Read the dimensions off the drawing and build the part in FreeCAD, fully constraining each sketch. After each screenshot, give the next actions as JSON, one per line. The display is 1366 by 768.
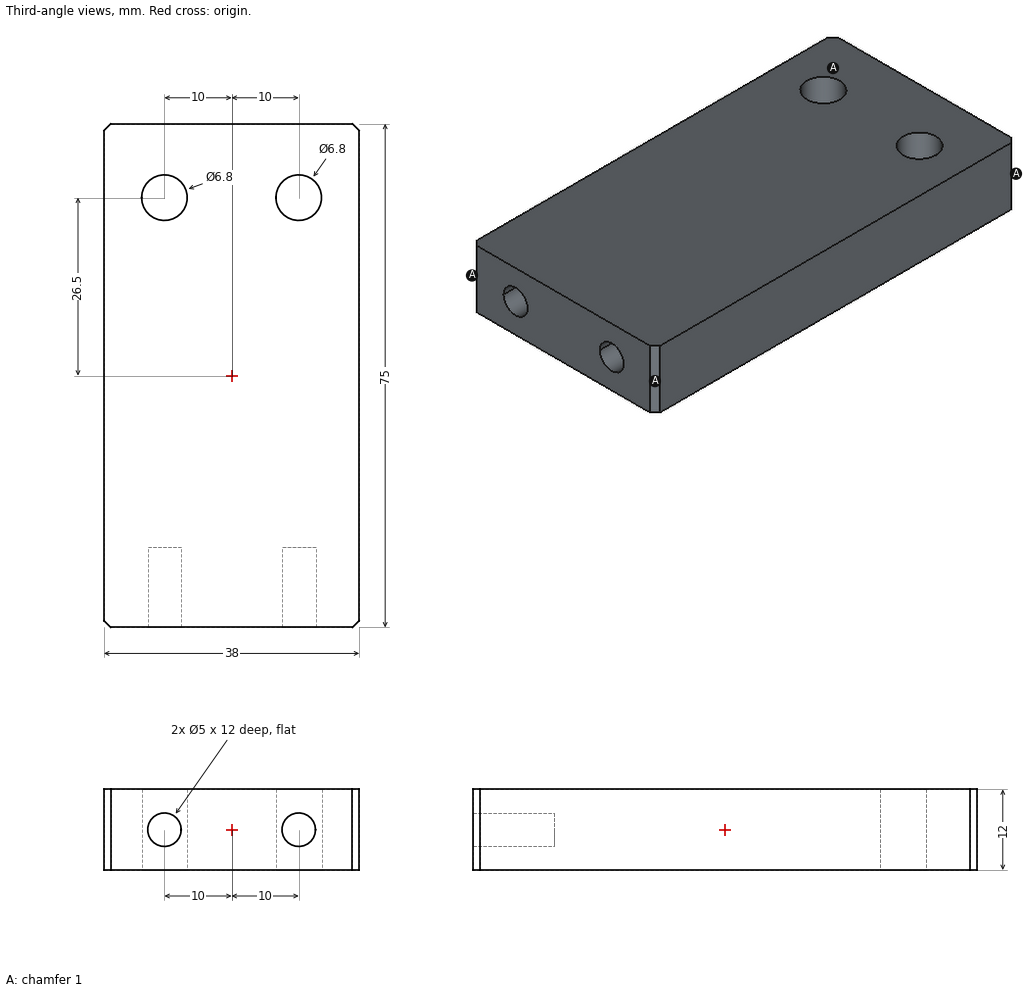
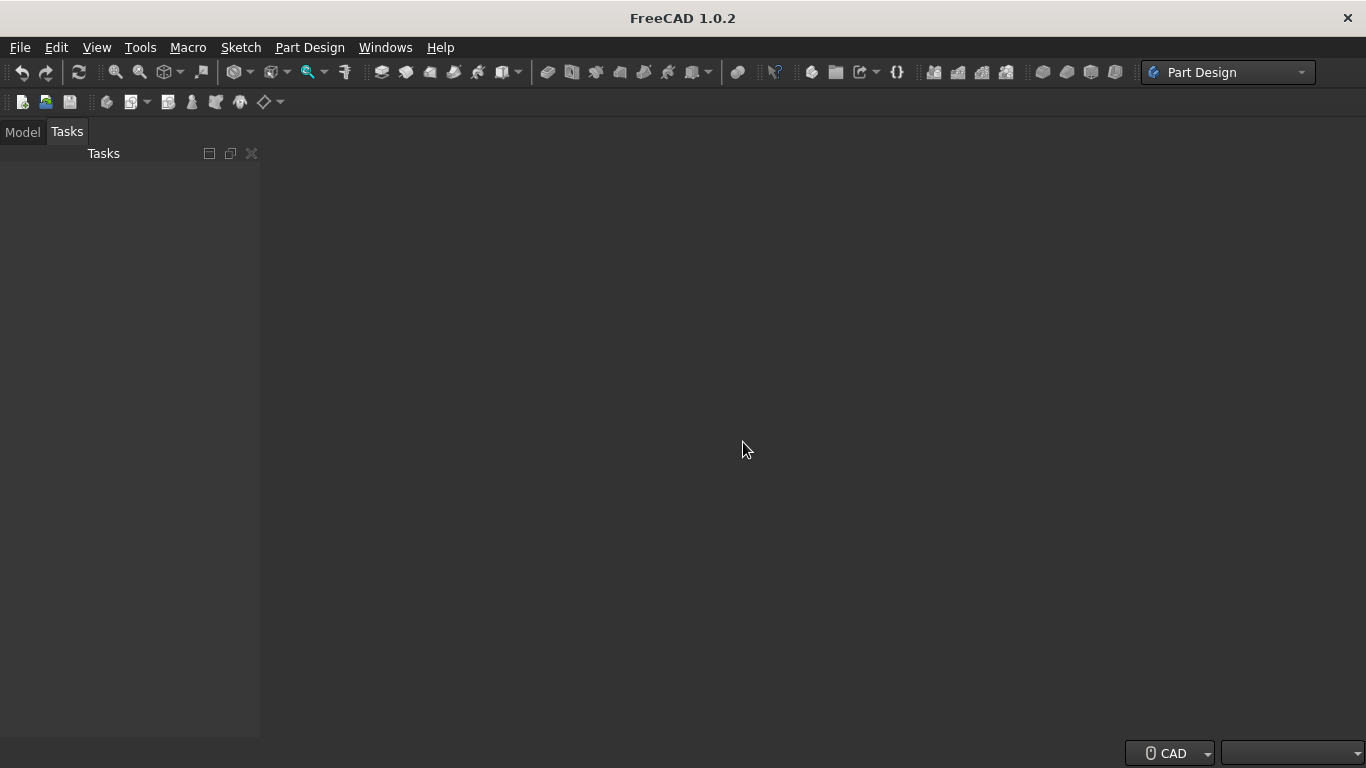
{"action": "key", "text": "ctrl+n"}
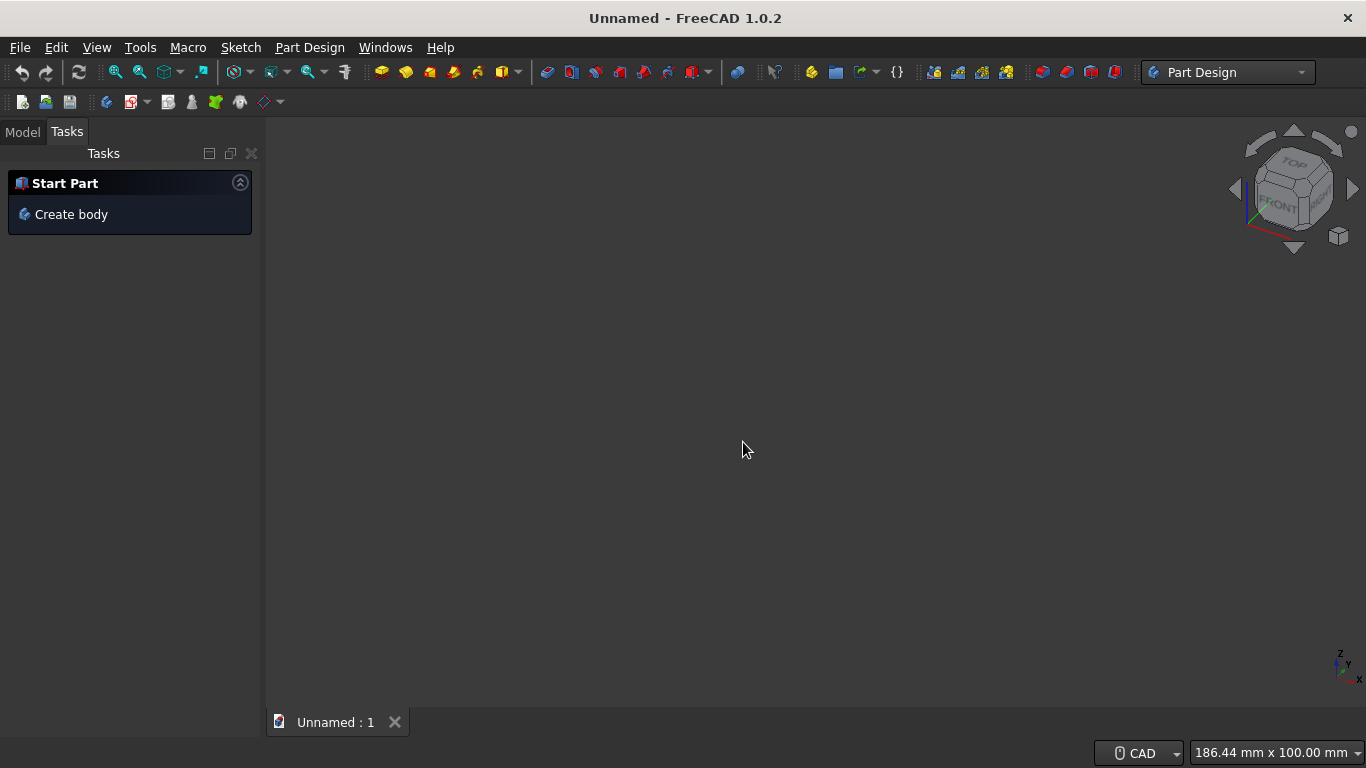
{"action": "left_click", "coordinate": [132, 102]}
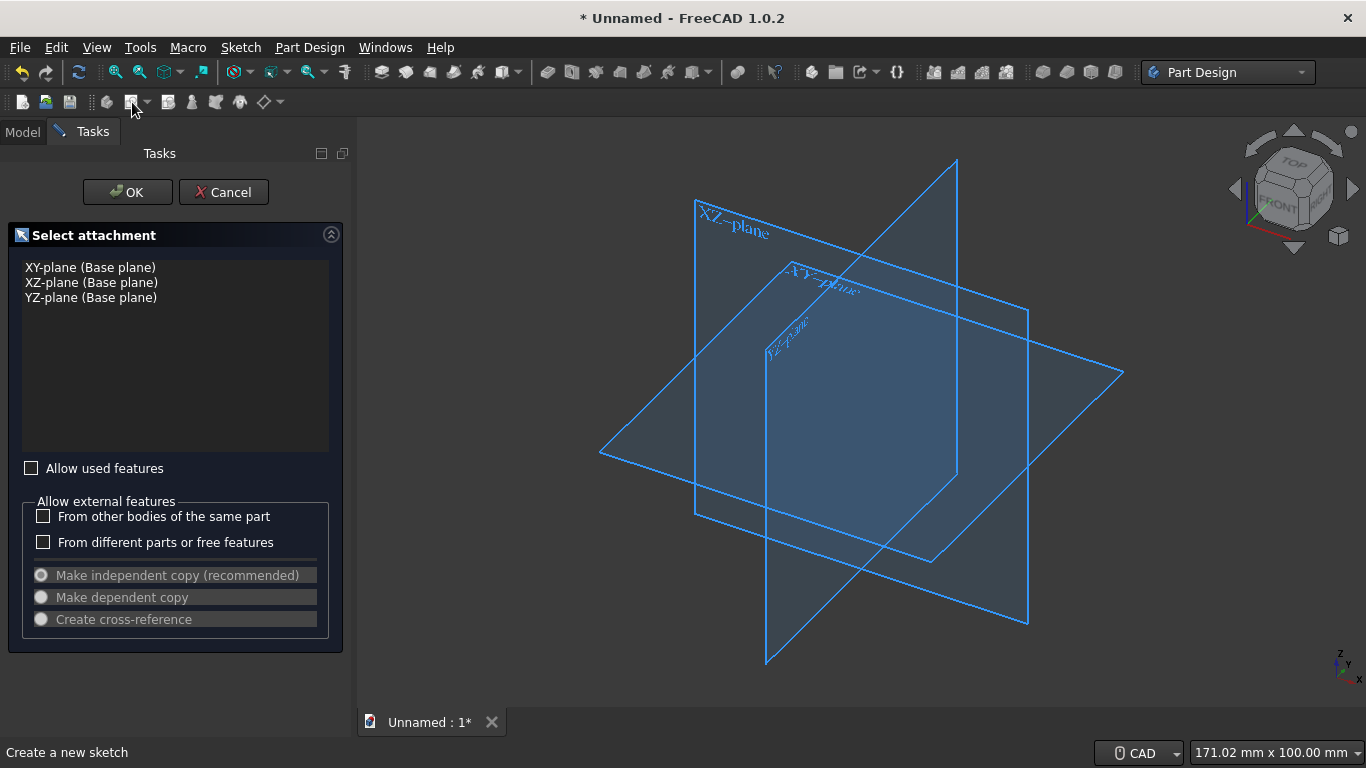
{"action": "left_click", "coordinate": [82, 268]}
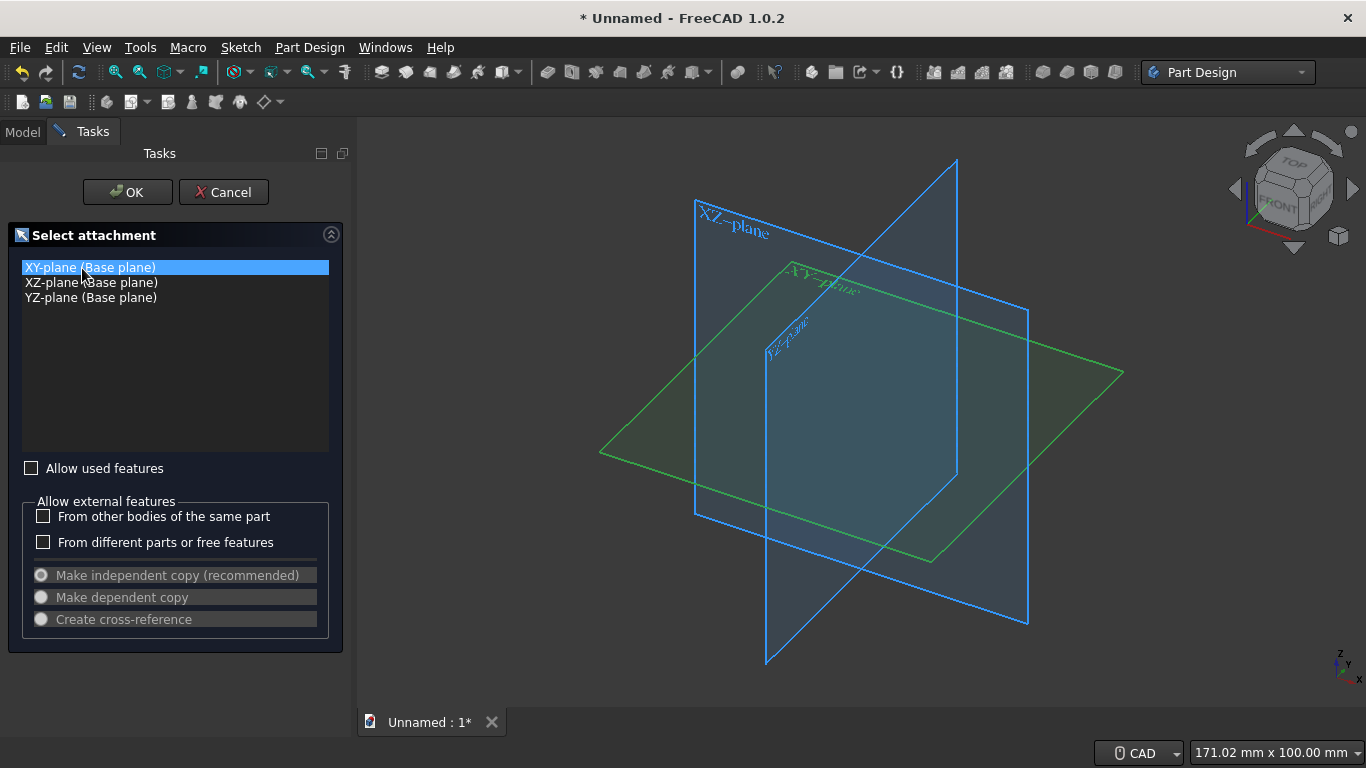
{"action": "left_click", "coordinate": [128, 192]}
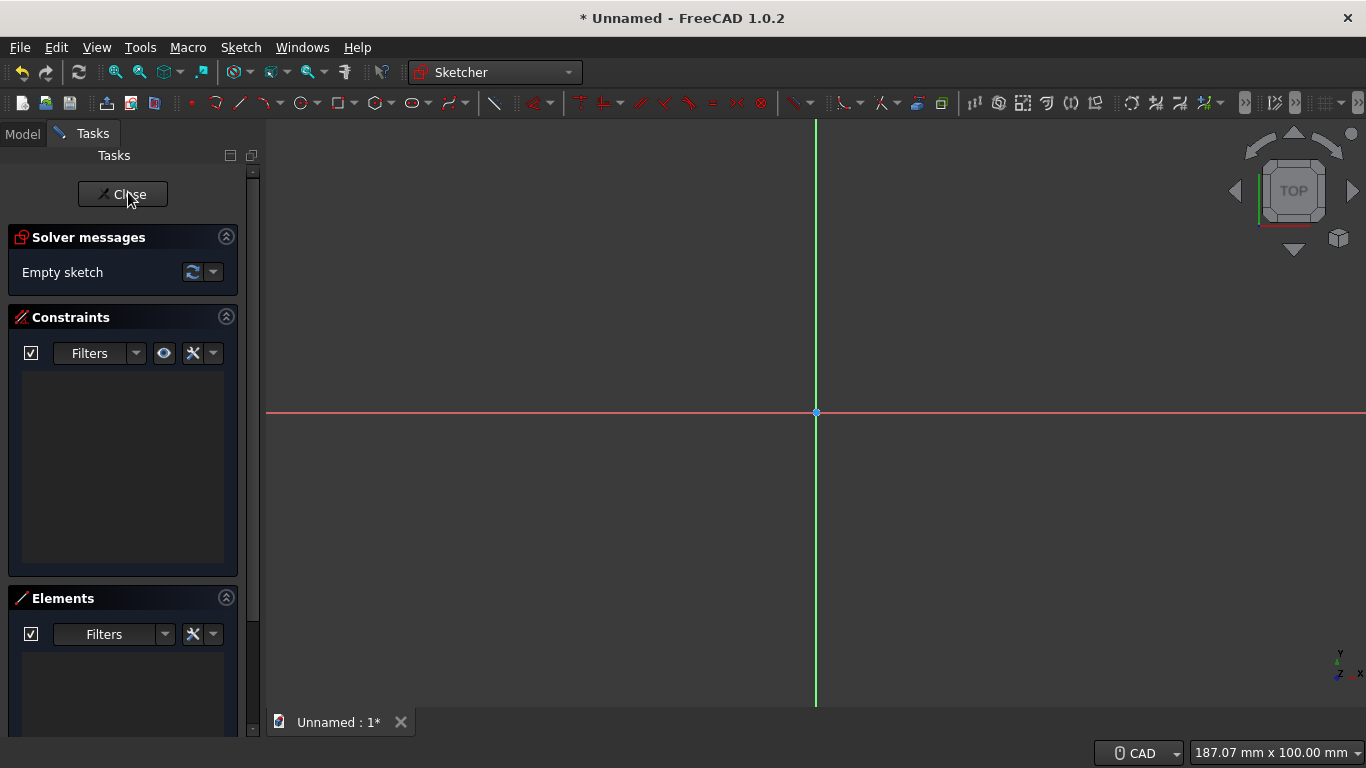
{"action": "key", "text": "g v"}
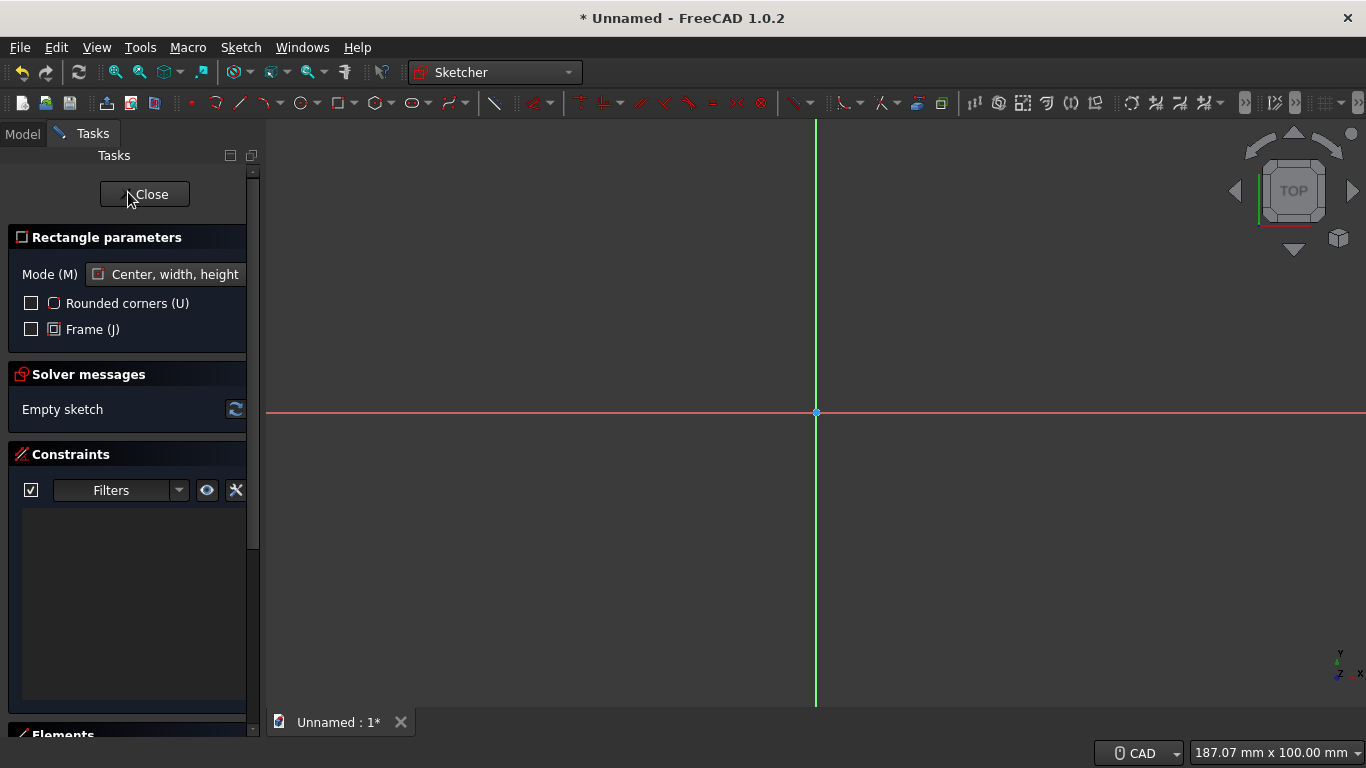
{"action": "left_click", "coordinate": [816, 413]}
{"action": "mouse_move", "coordinate": [928, 192]}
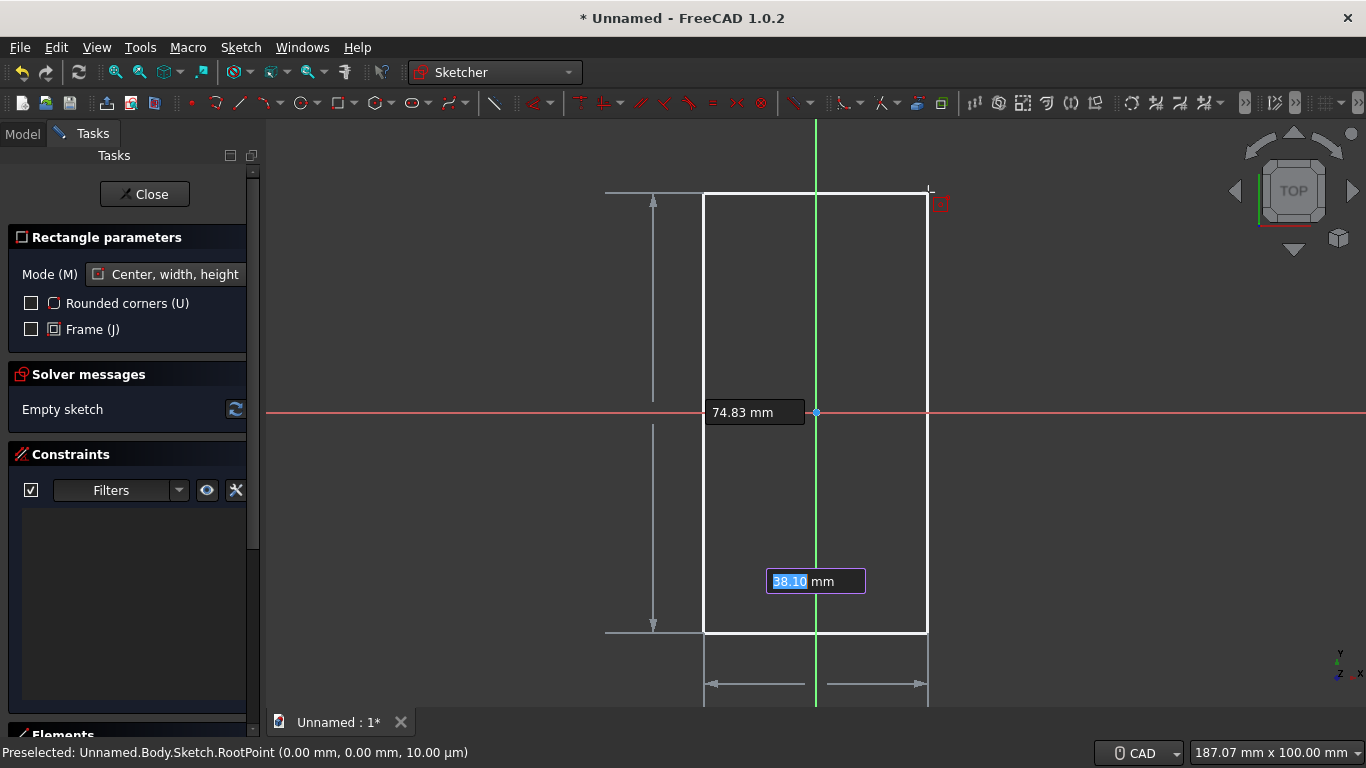
{"action": "type", "text": "38"}
{"action": "key", "text": "Tab"}
{"action": "type", "text": "75"}
{"action": "key", "text": "Return"}
{"action": "key", "text": "Escape"}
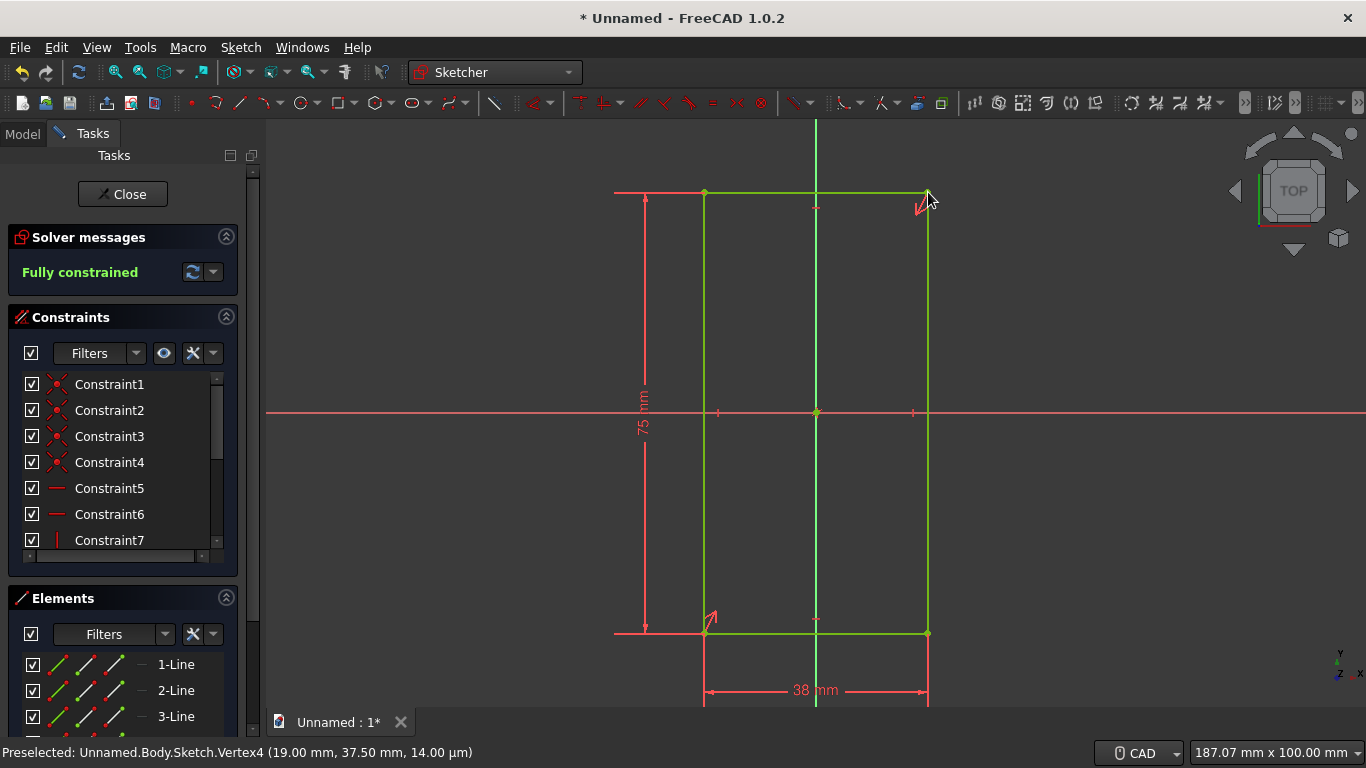
{"action": "left_click", "coordinate": [123, 194]}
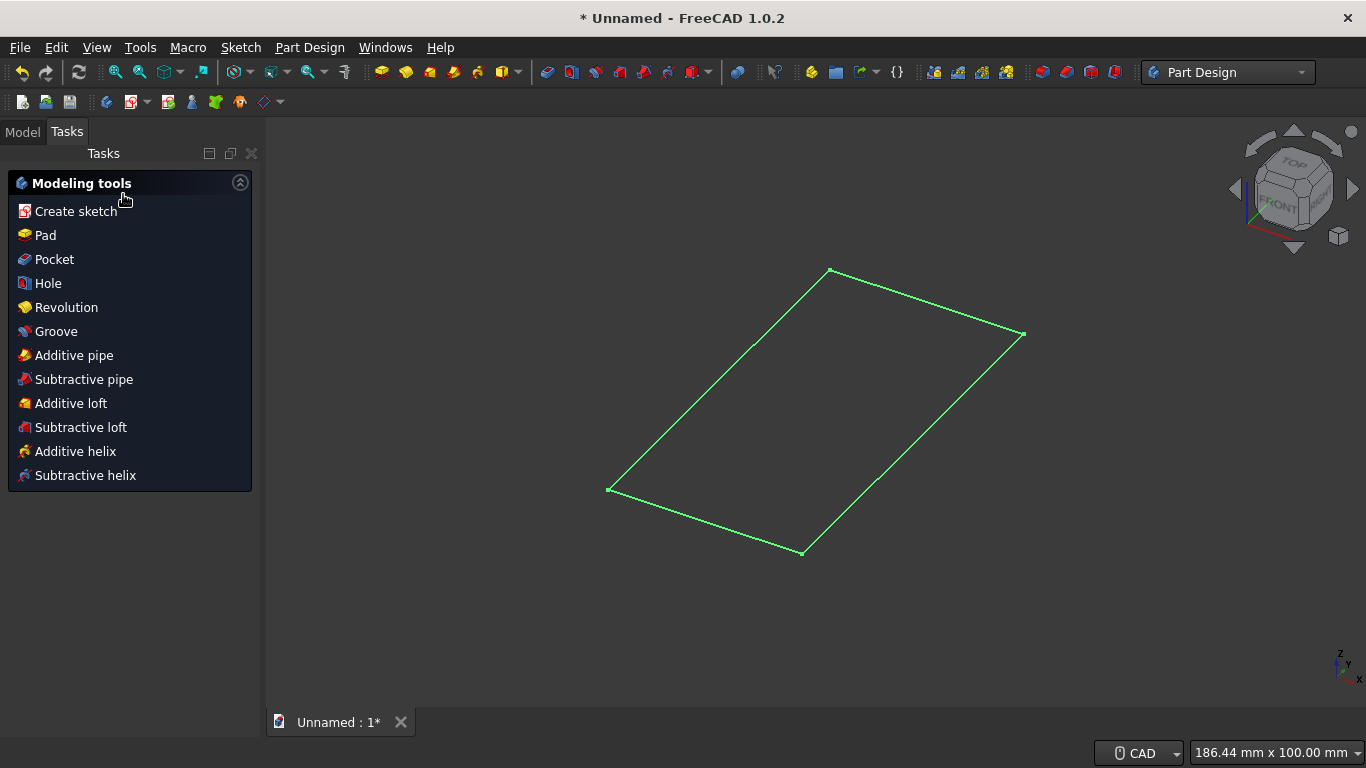
{"action": "left_click", "coordinate": [382, 72]}